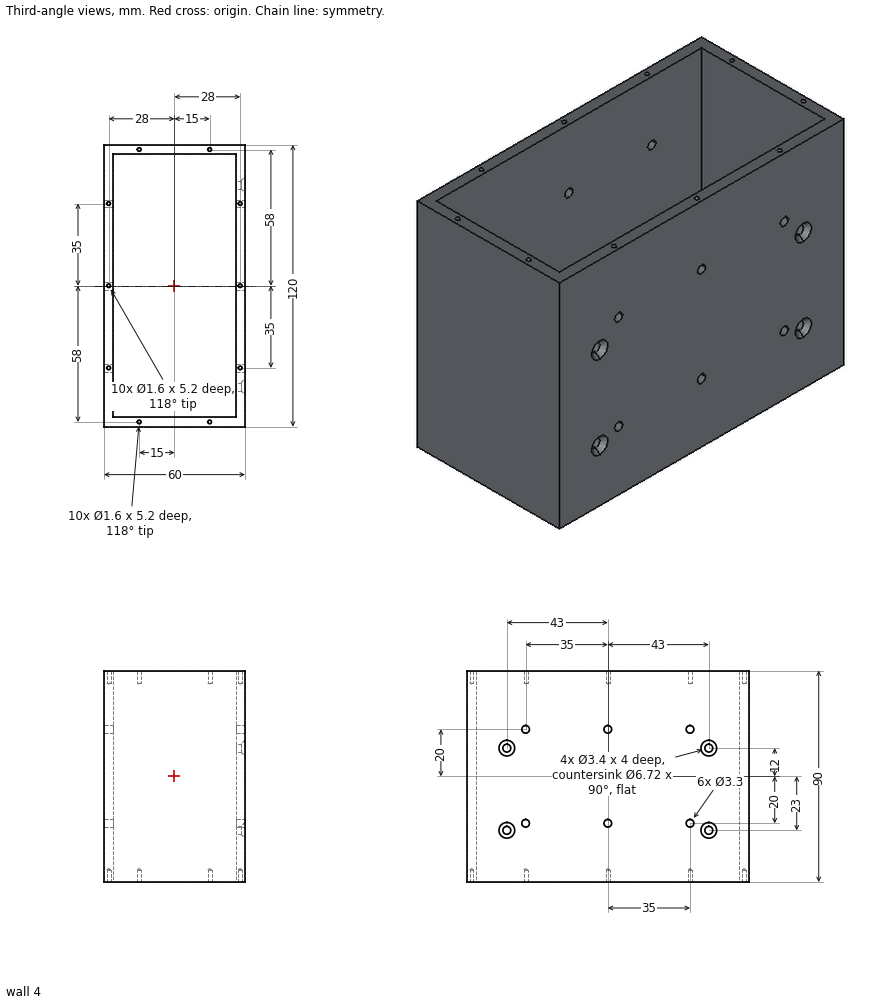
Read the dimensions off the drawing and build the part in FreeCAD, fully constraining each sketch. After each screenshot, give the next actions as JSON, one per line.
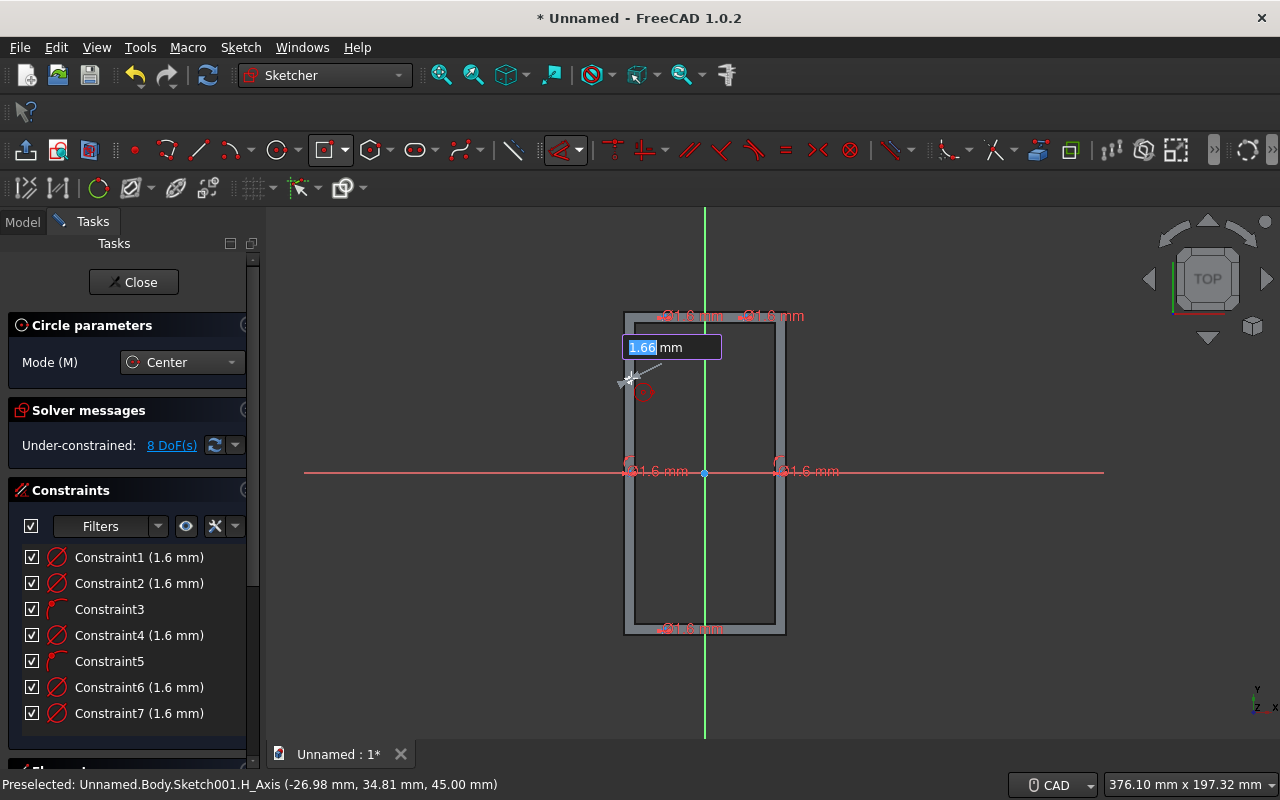
{"action": "type", "text": "1.6"}
{"action": "key", "text": "Return"}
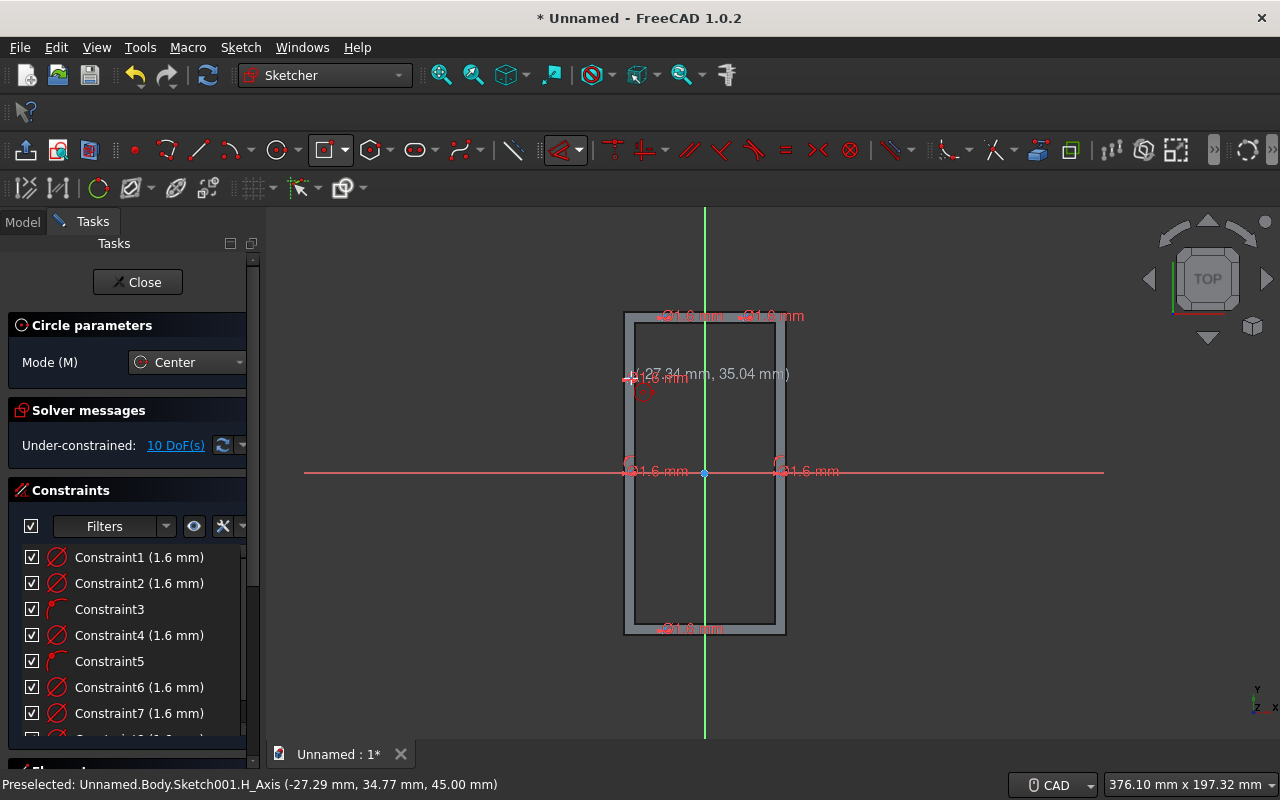
{"action": "scroll", "coordinate": [780, 379], "scroll_direction": "up", "scroll_amount": 12}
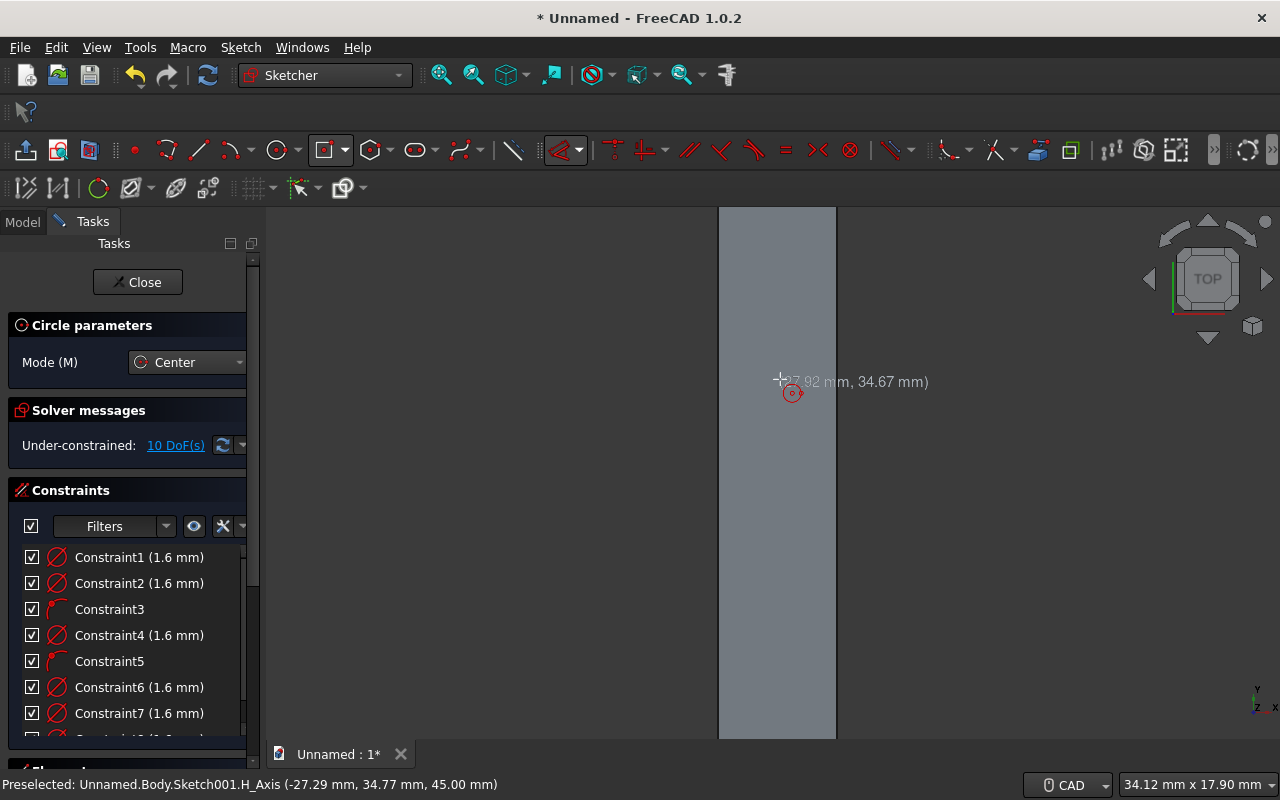
{"action": "scroll", "coordinate": [780, 379], "scroll_direction": "down", "scroll_amount": 12}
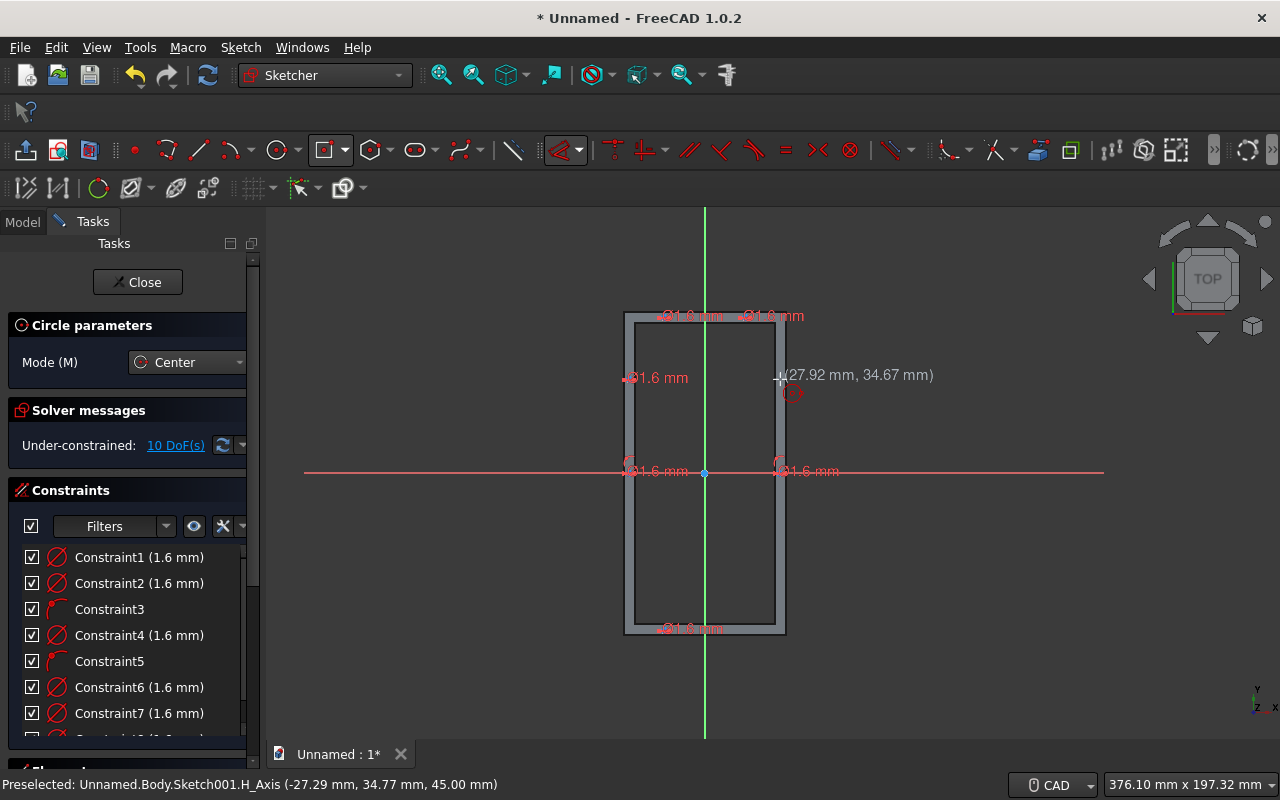
{"action": "left_click", "coordinate": [780, 379]}
{"action": "mouse_move", "coordinate": [782, 378]}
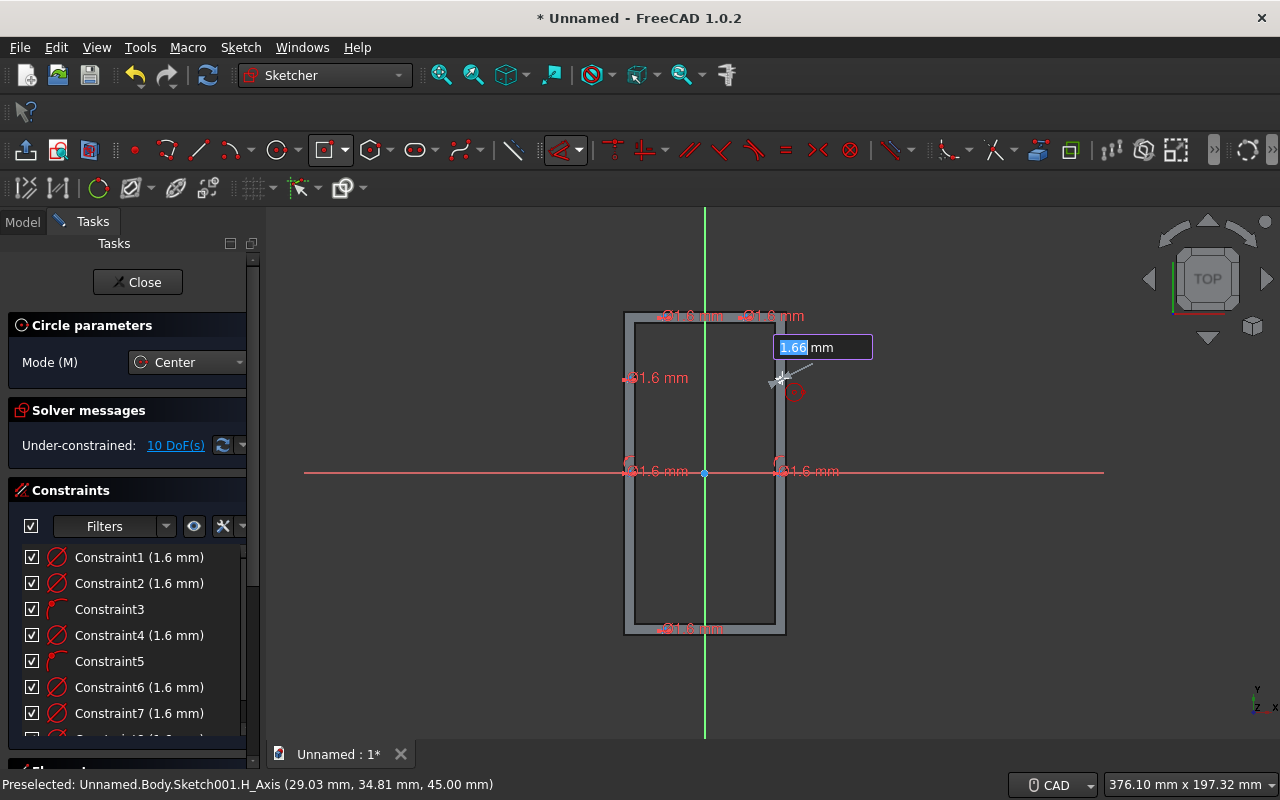
{"action": "type", "text": "1.6"}
{"action": "key", "text": "Return"}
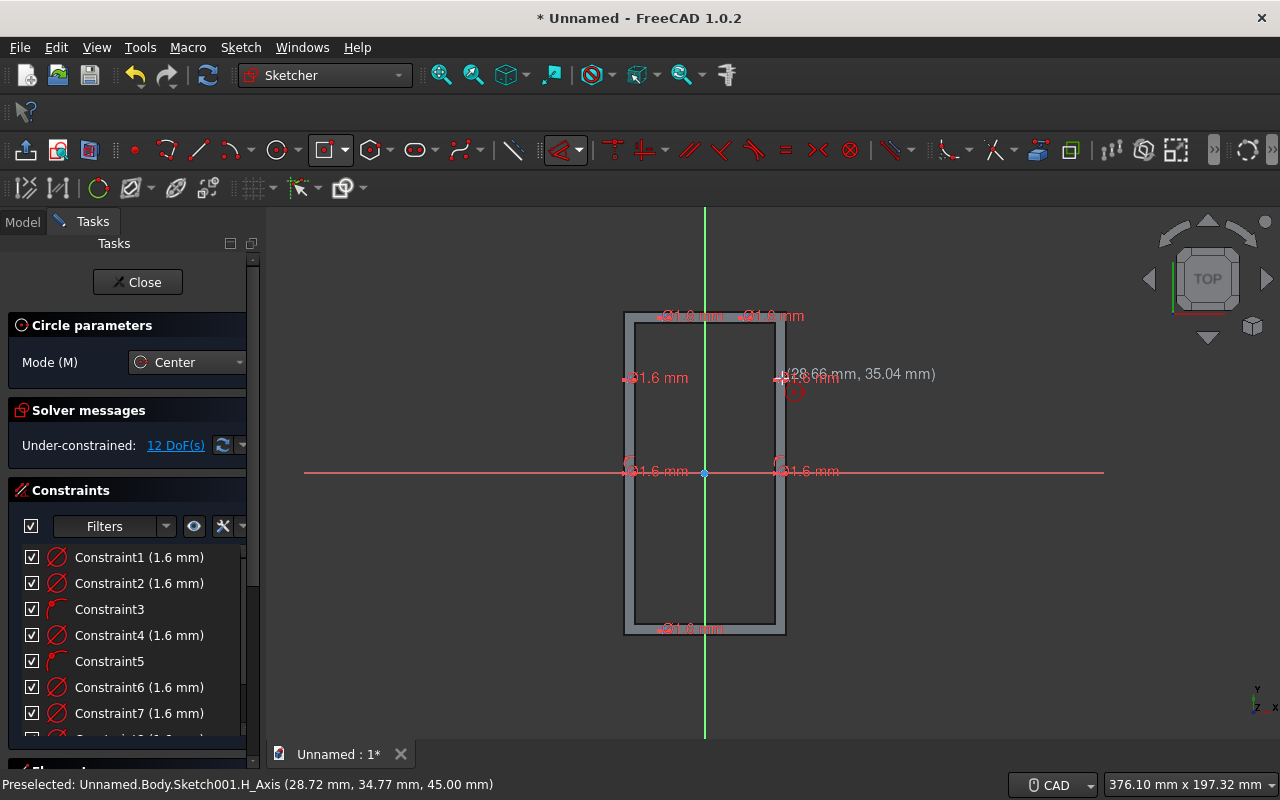
{"action": "scroll", "coordinate": [780, 568], "scroll_direction": "up", "scroll_amount": 12}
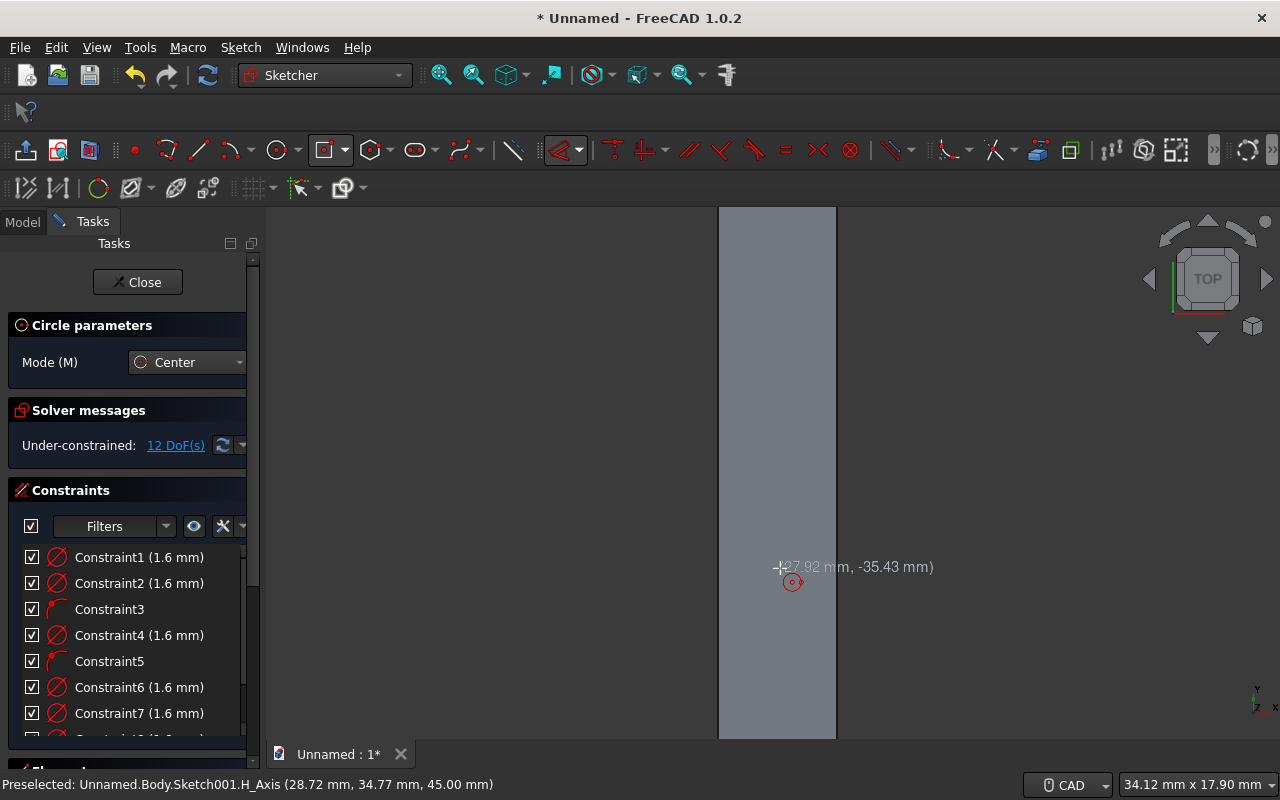
{"action": "scroll", "coordinate": [780, 568], "scroll_direction": "down", "scroll_amount": 12}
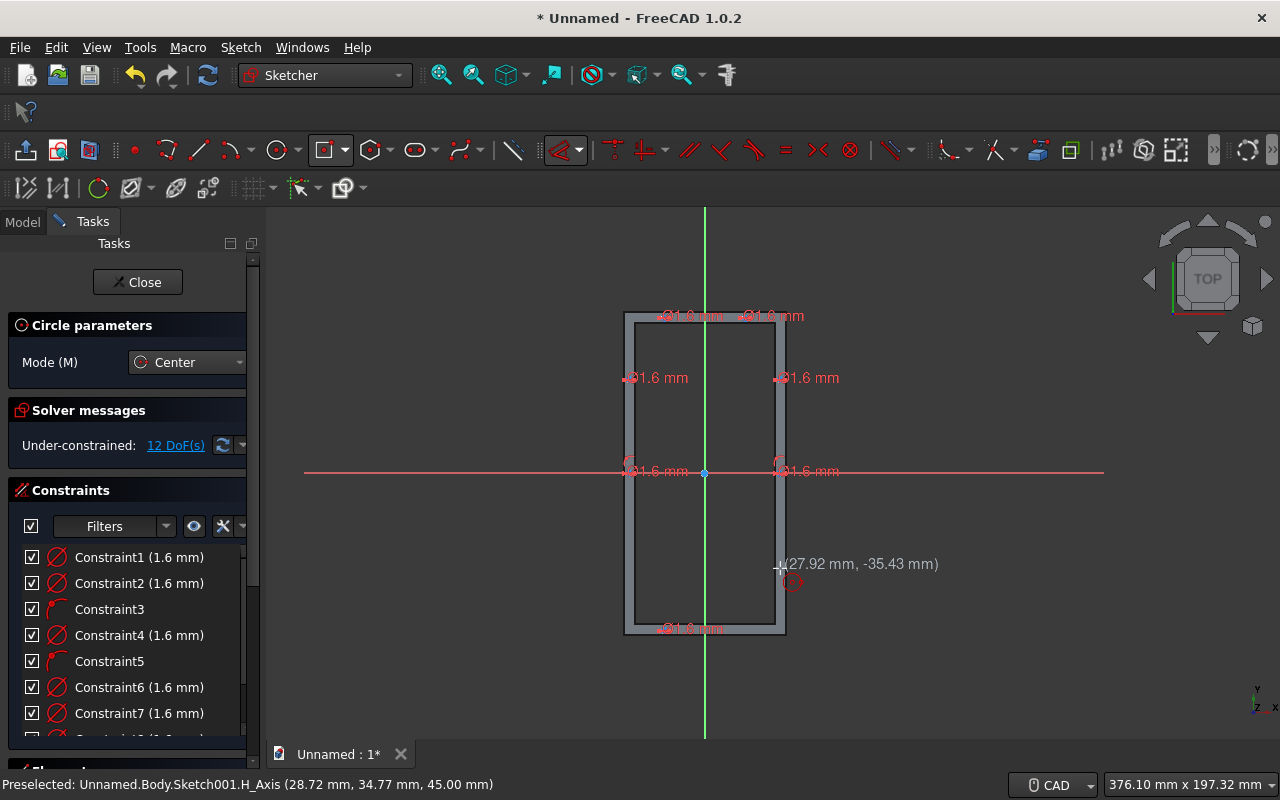
{"action": "left_click", "coordinate": [780, 568]}
{"action": "mouse_move", "coordinate": [782, 566]}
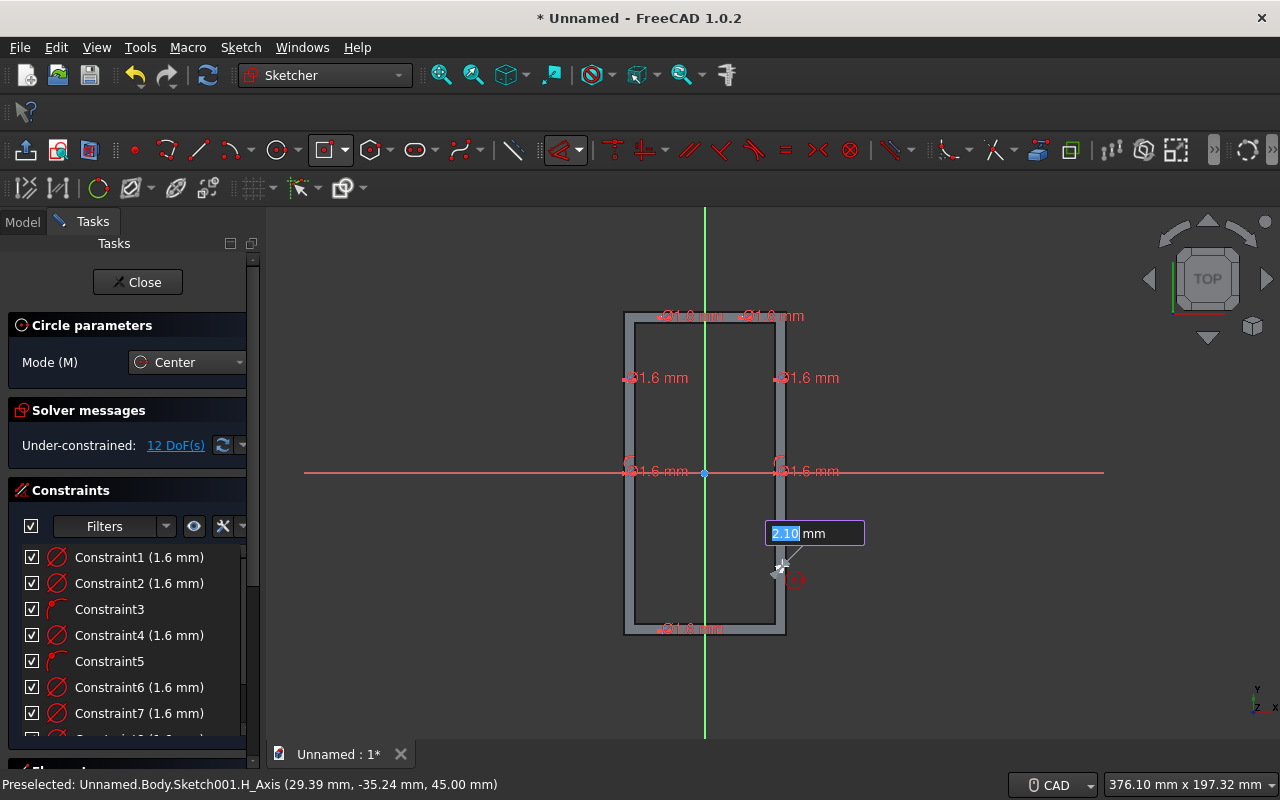
{"action": "type", "text": "1.6"}
{"action": "key", "text": "Return"}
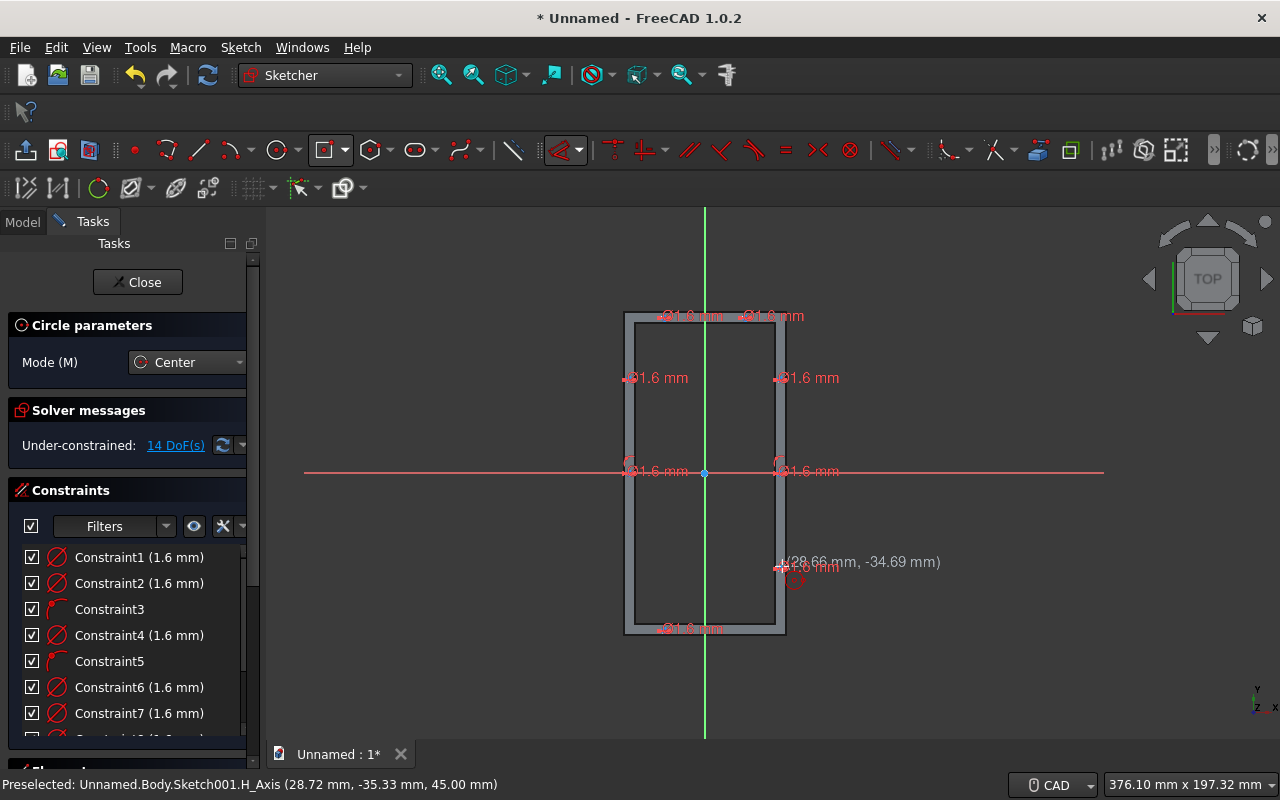
{"action": "scroll", "coordinate": [629, 568], "scroll_direction": "up", "scroll_amount": 12}